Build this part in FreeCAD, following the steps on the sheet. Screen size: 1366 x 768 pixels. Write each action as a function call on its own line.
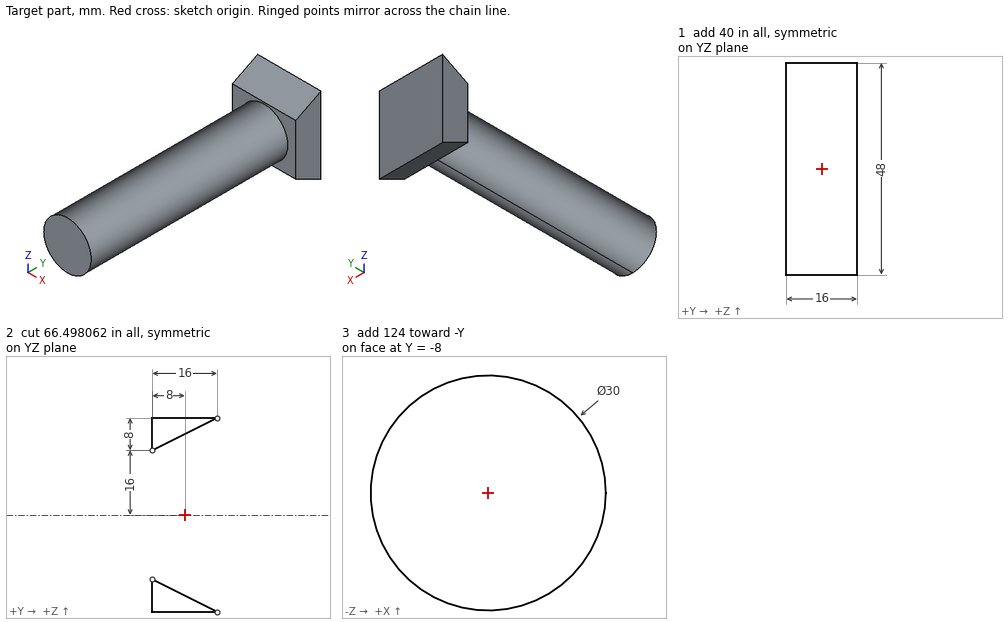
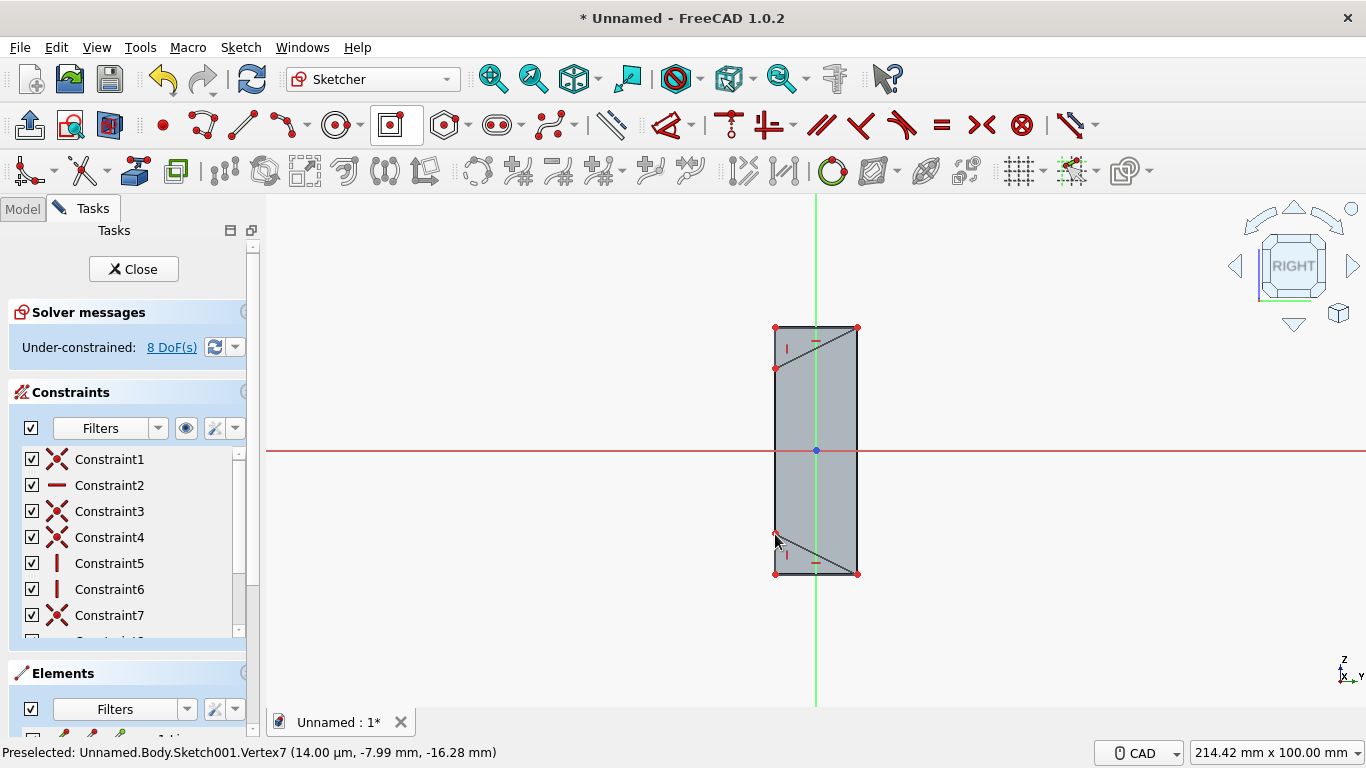
click(775, 369)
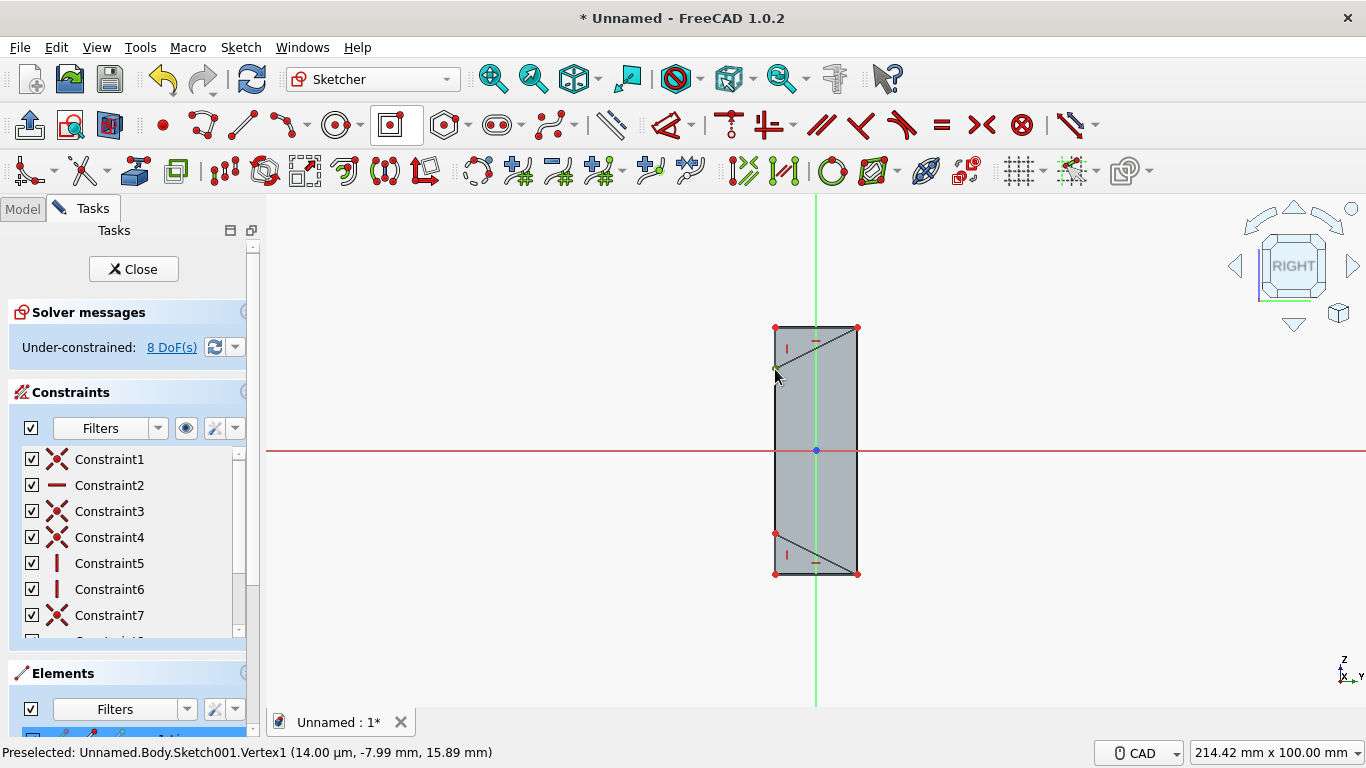
click(775, 534)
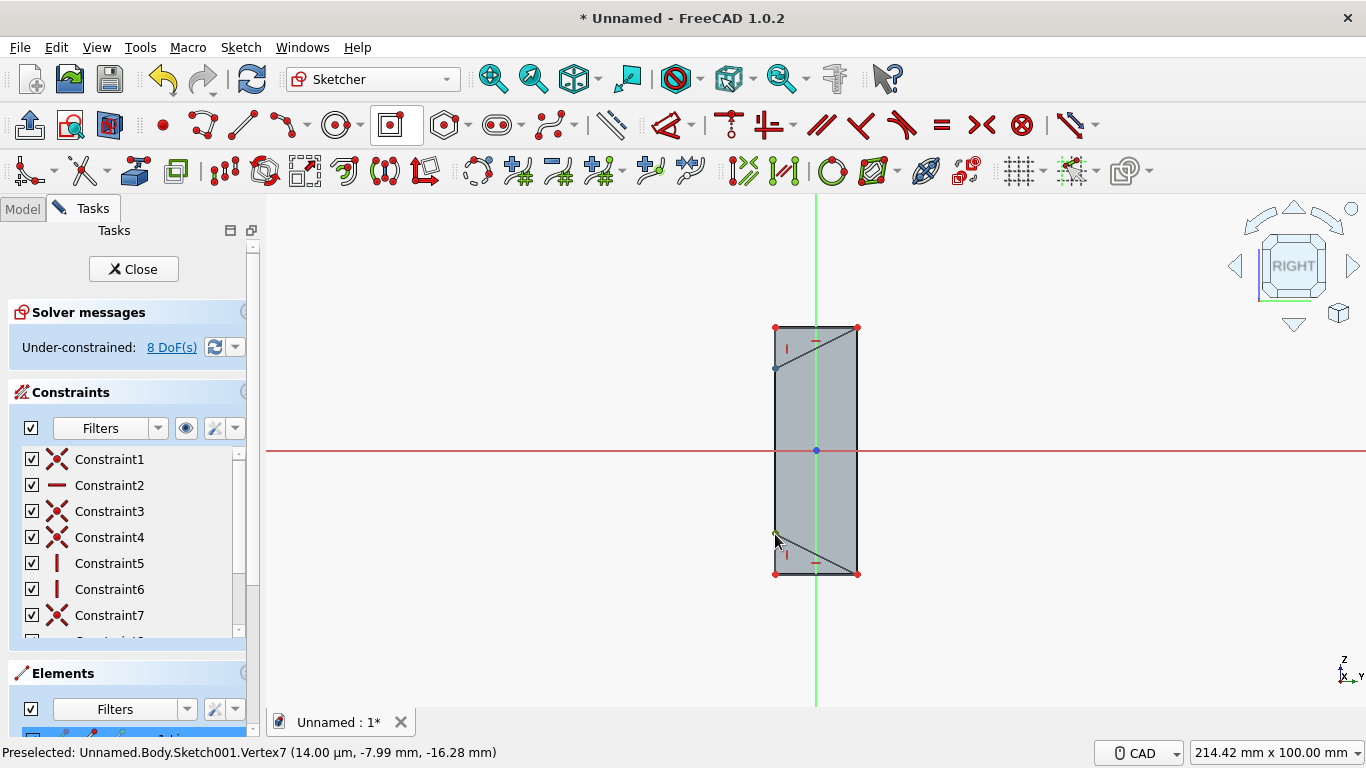
click(359, 450)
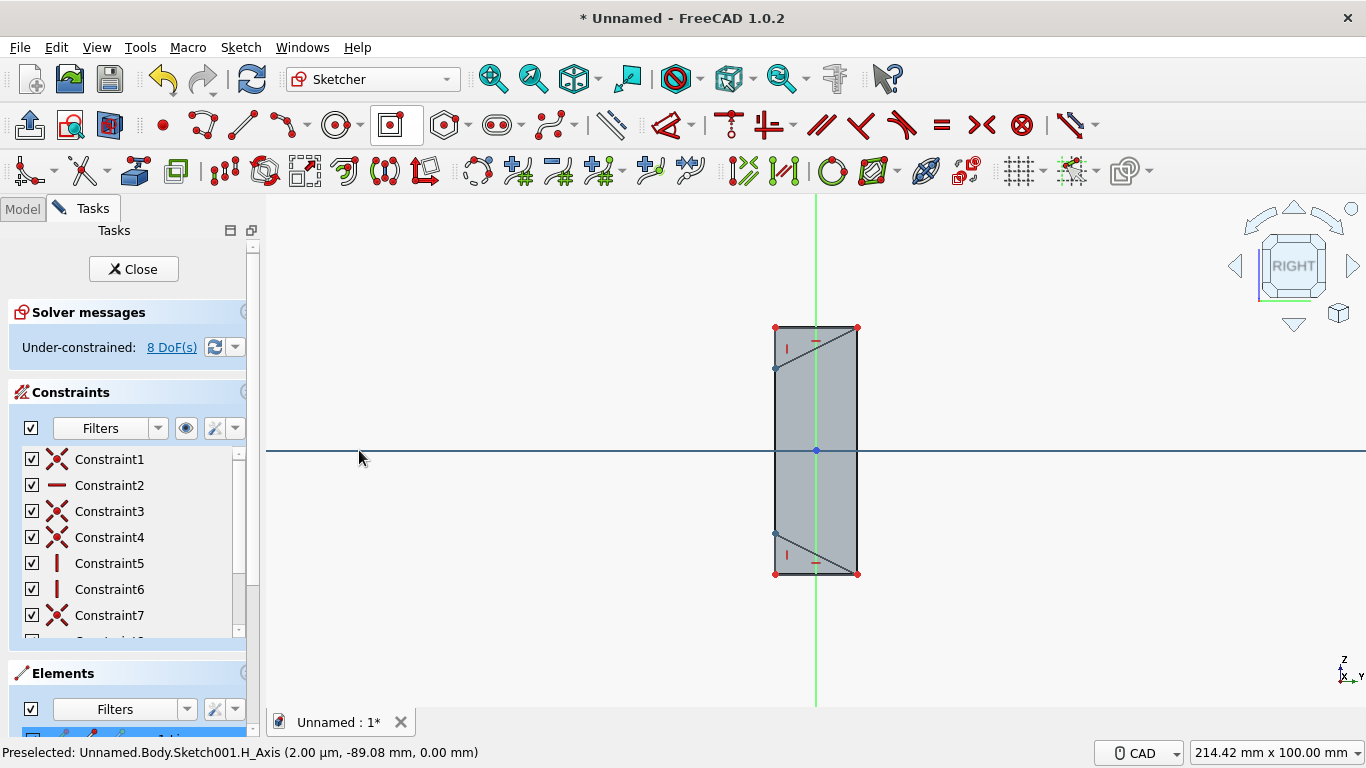
click(982, 126)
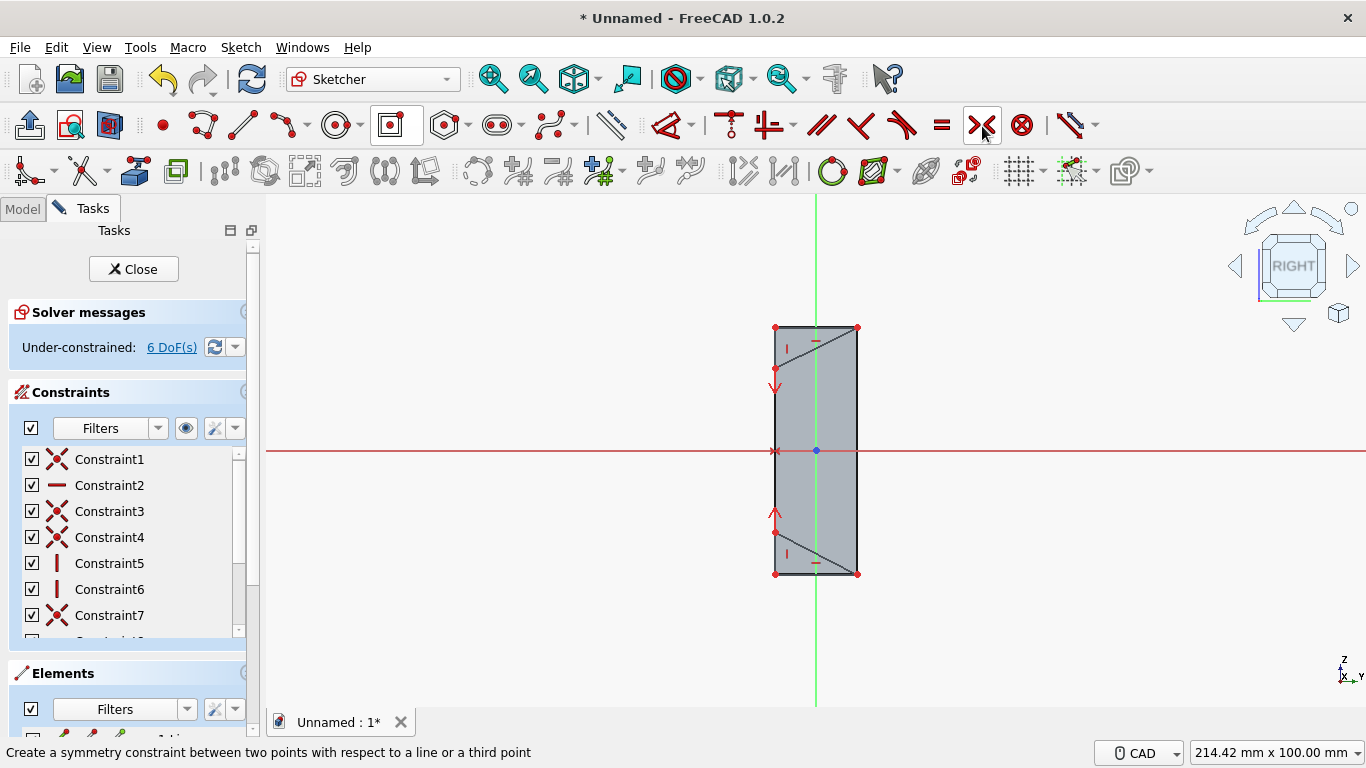
click(857, 328)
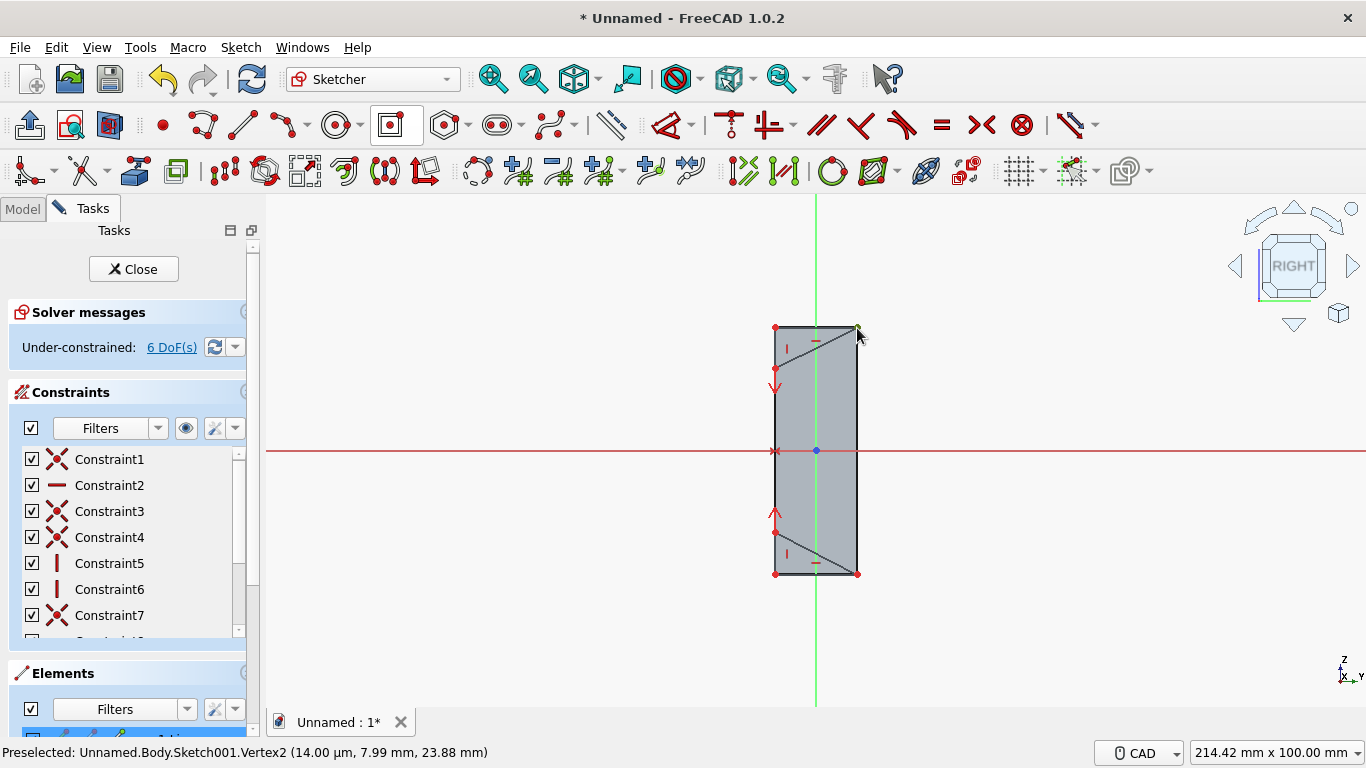
click(857, 575)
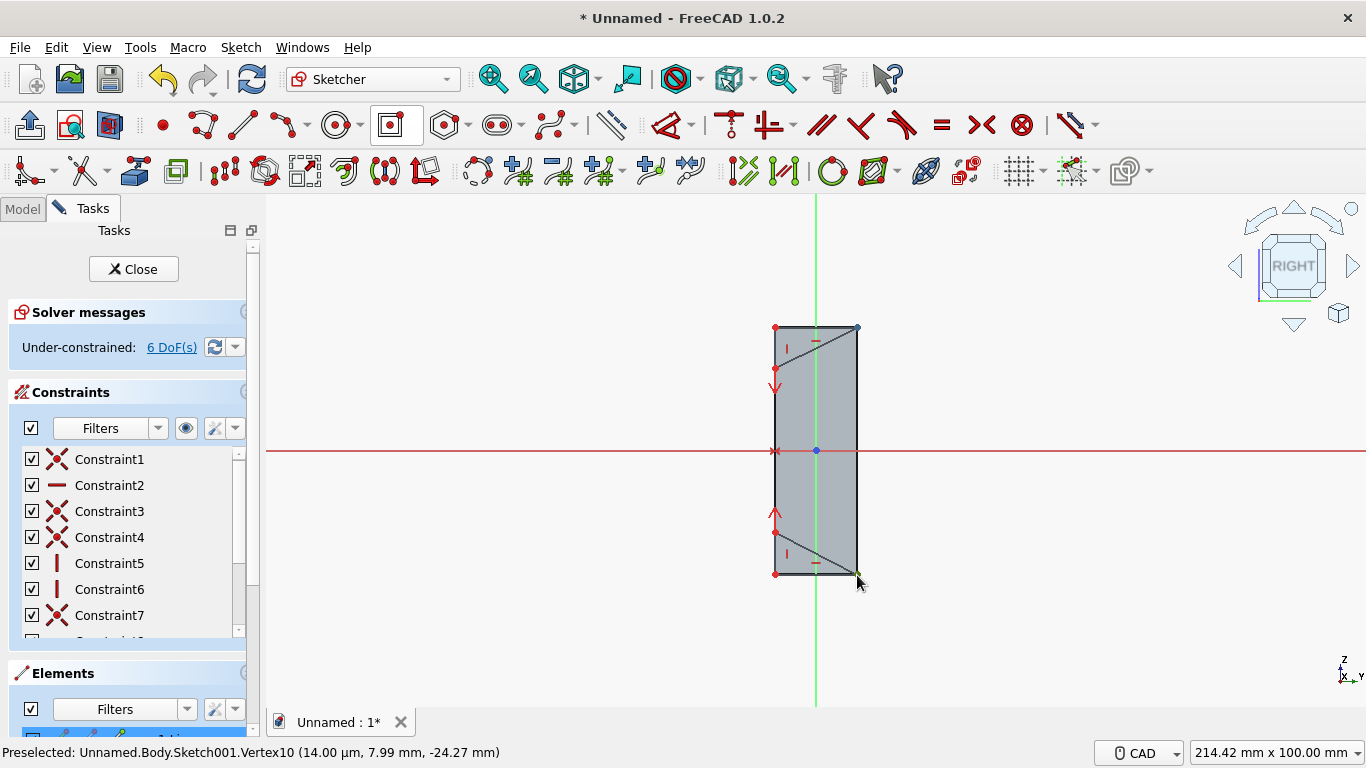
click(359, 450)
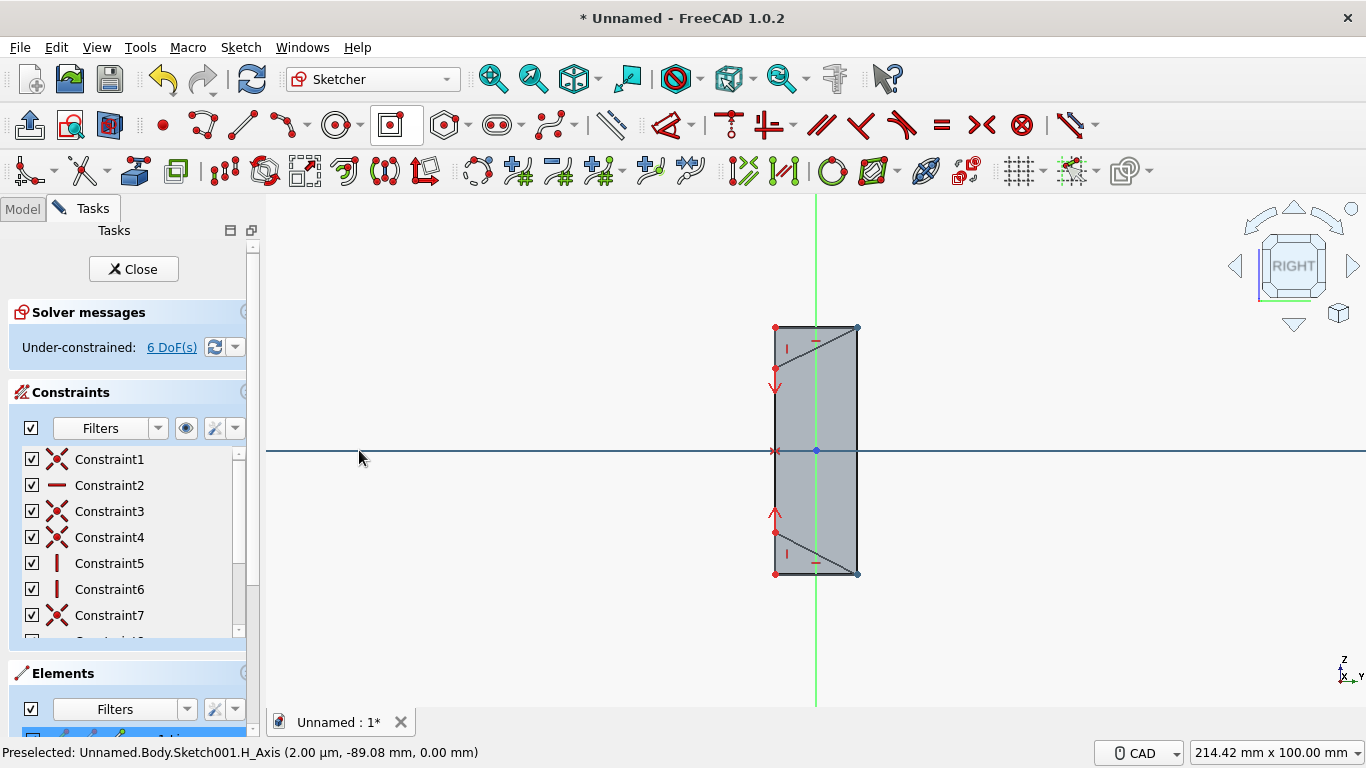
click(982, 126)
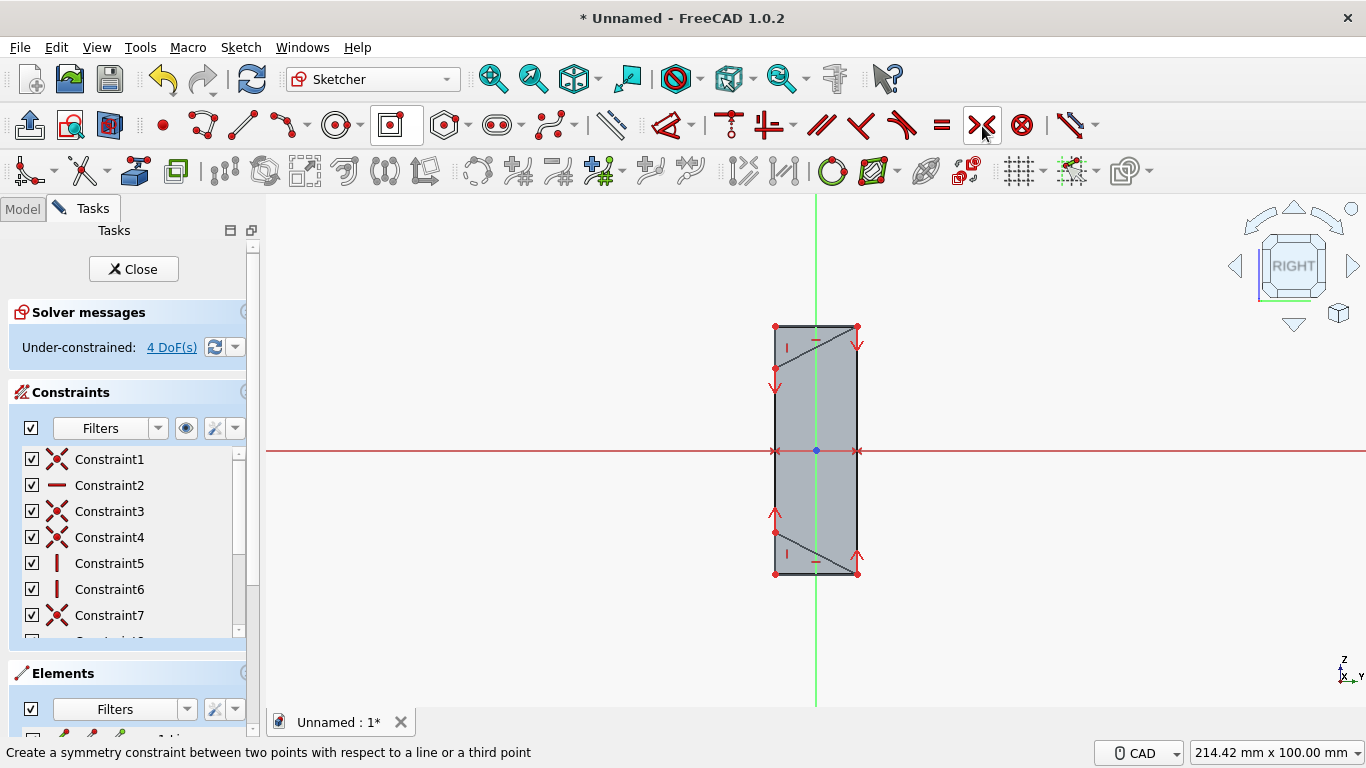
click(775, 339)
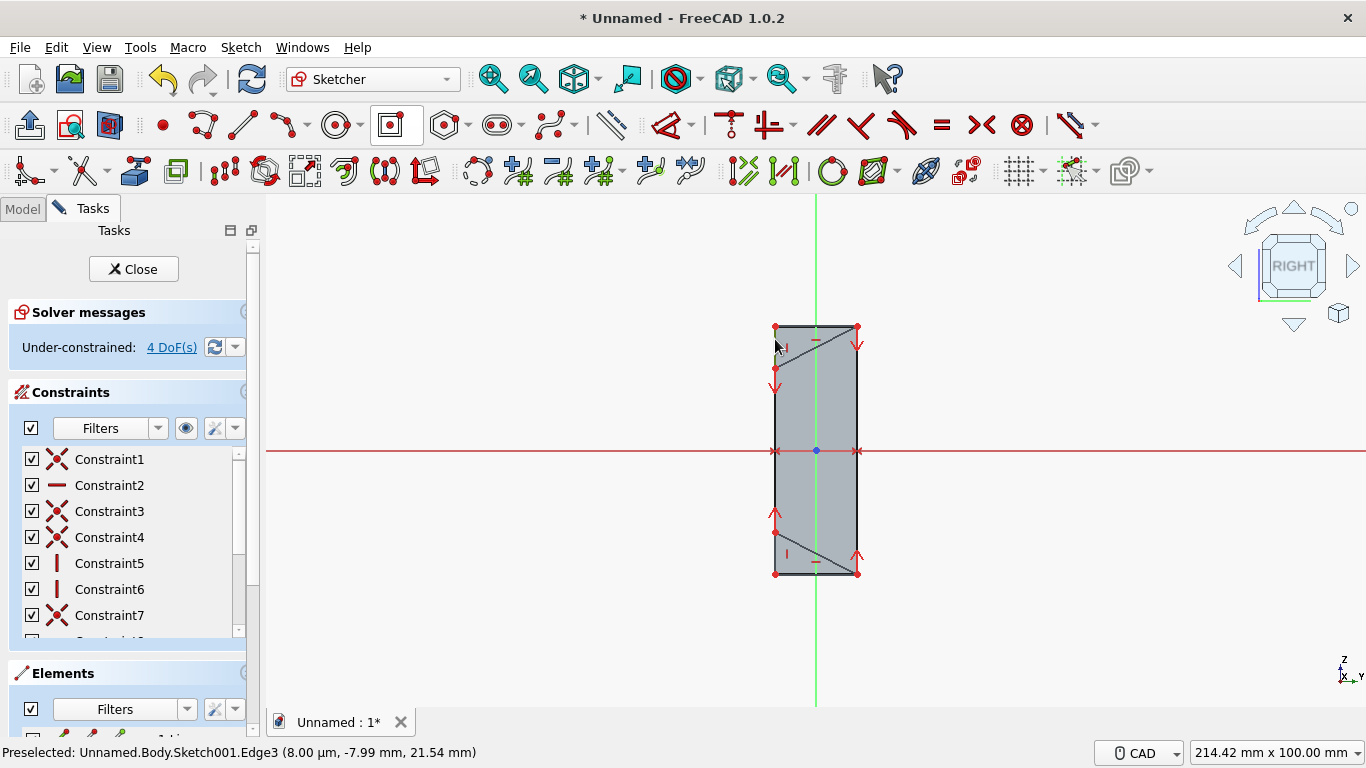
key(i)